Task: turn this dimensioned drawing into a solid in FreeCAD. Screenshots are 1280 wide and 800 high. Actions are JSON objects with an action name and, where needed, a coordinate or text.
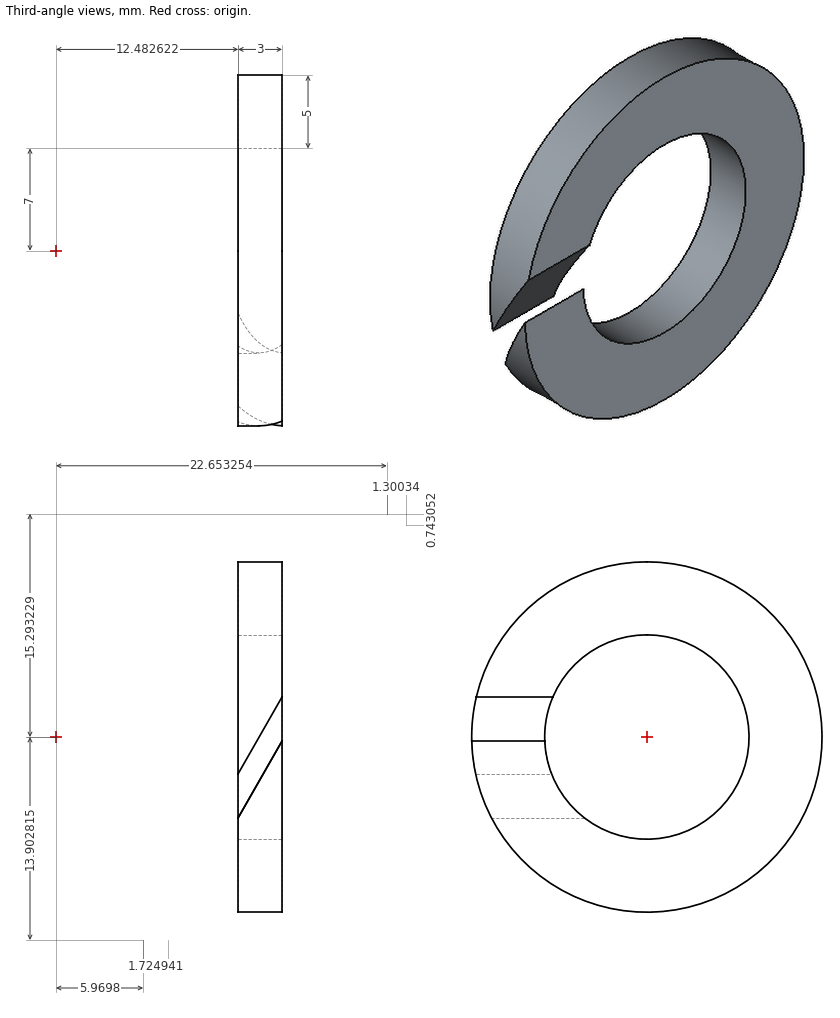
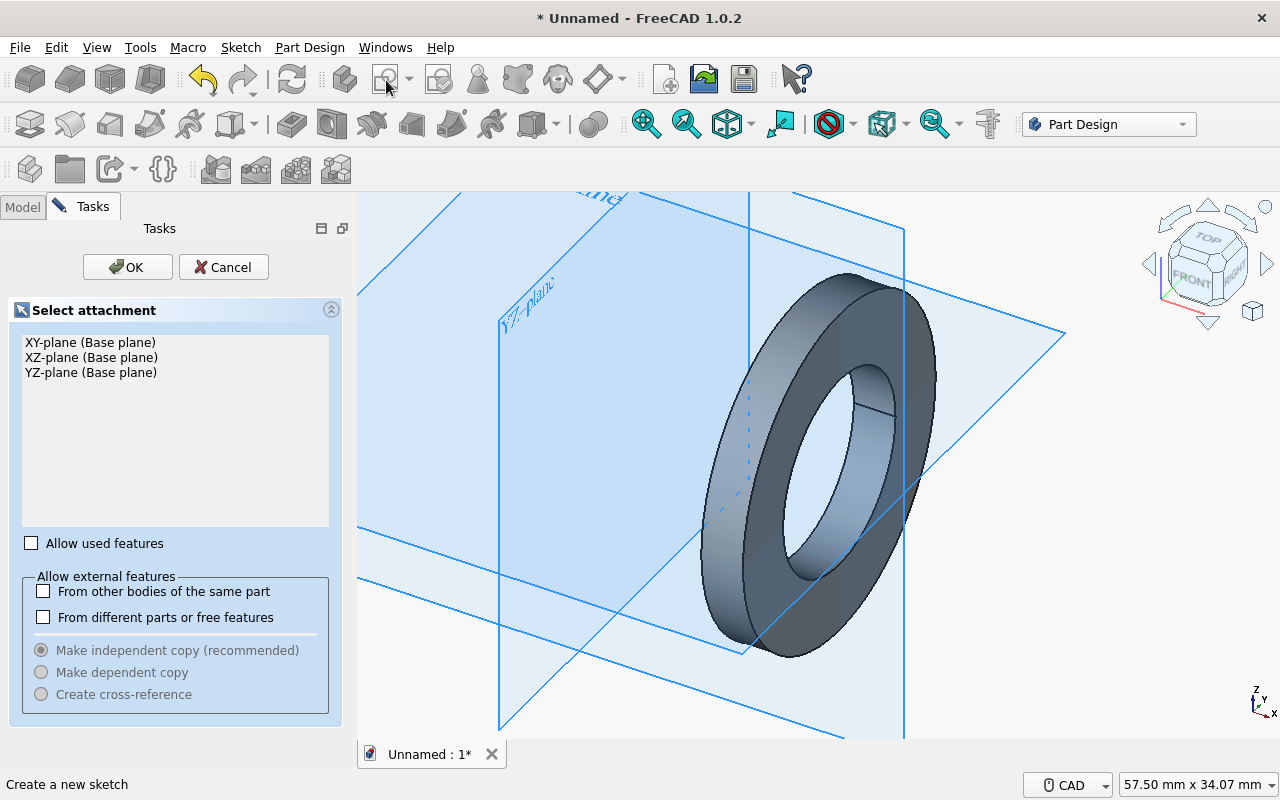
{"action": "left_click", "coordinate": [82, 358]}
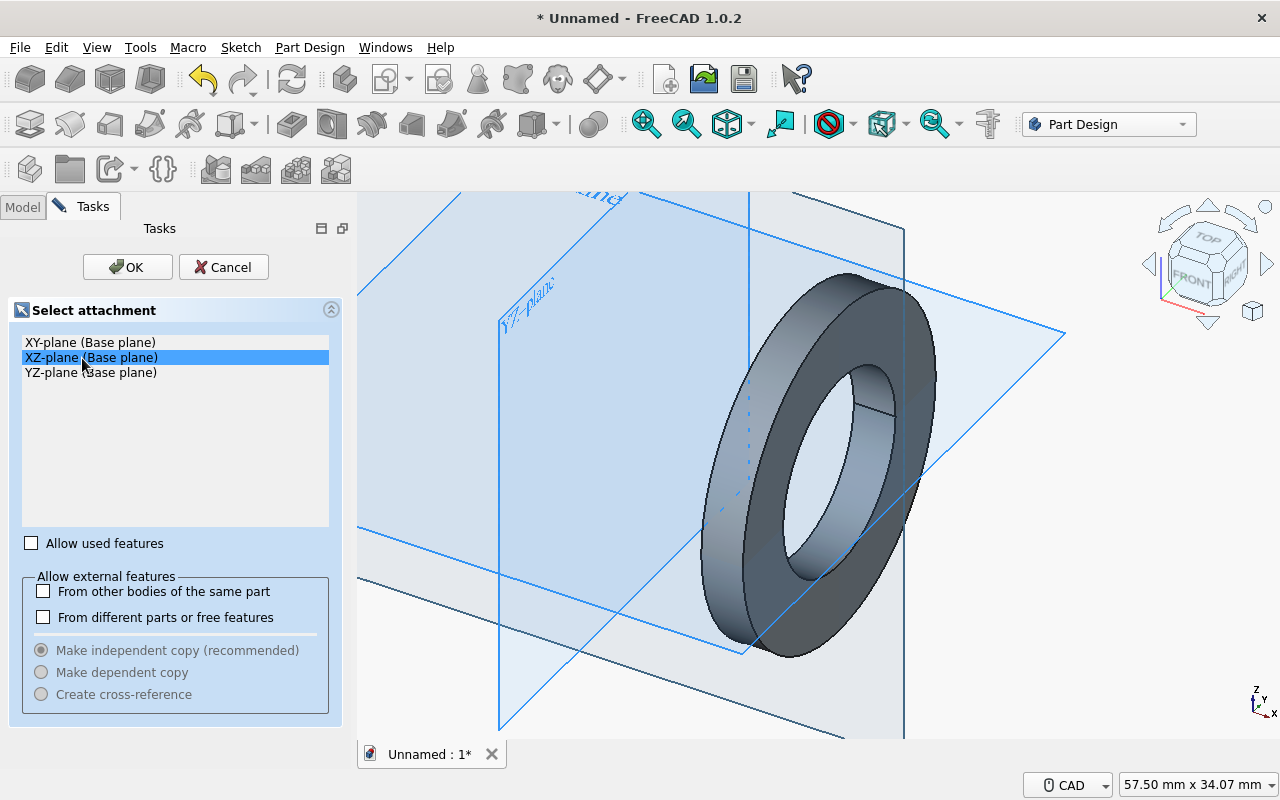
{"action": "left_click", "coordinate": [128, 267]}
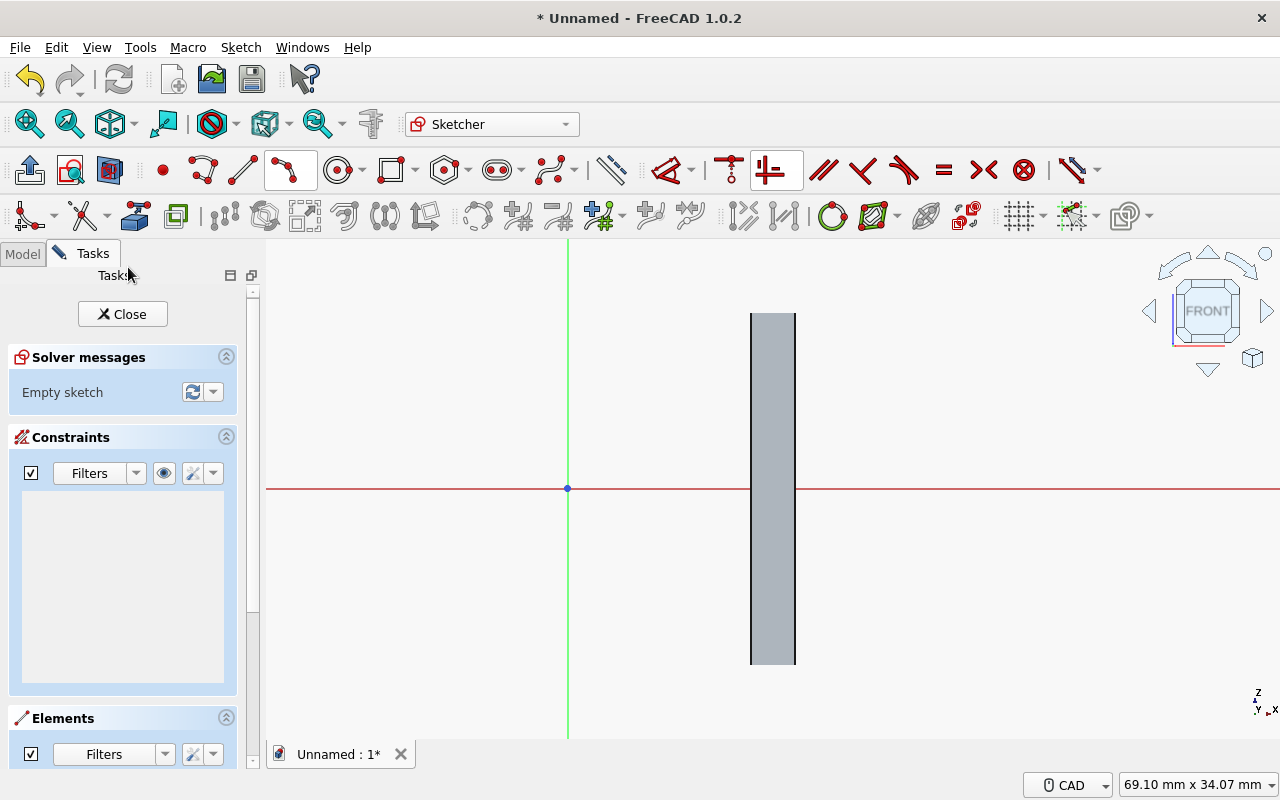
{"action": "key", "text": "q s"}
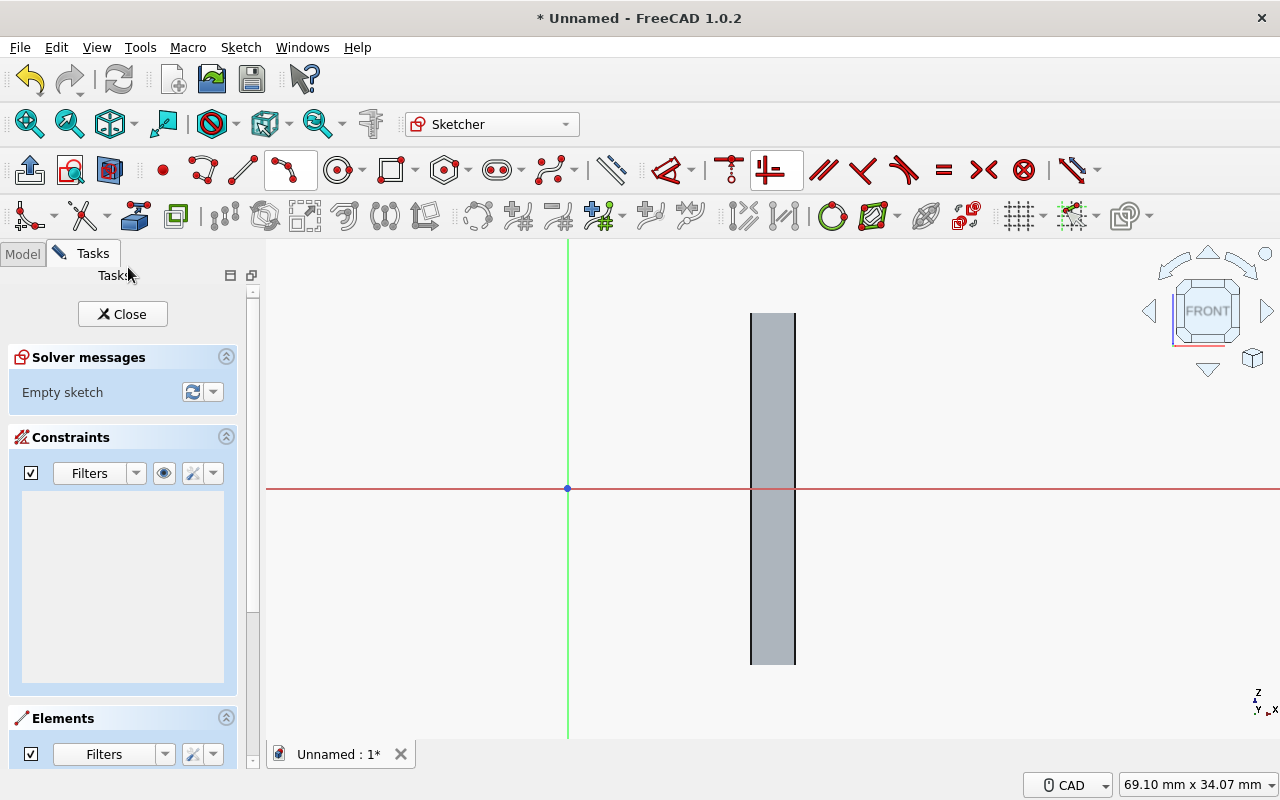
{"action": "scroll", "coordinate": [625, 510], "scroll_direction": "down", "scroll_amount": 2}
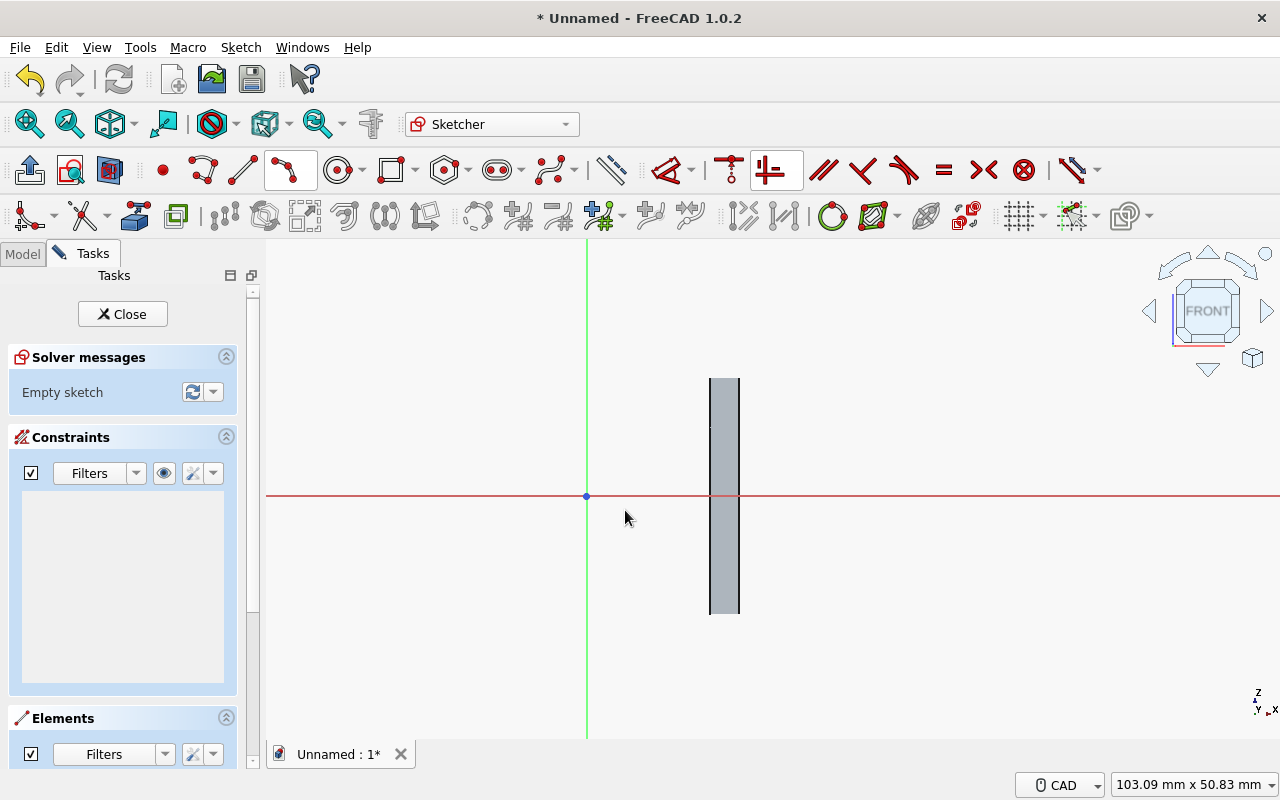
{"action": "key", "text": "g m"}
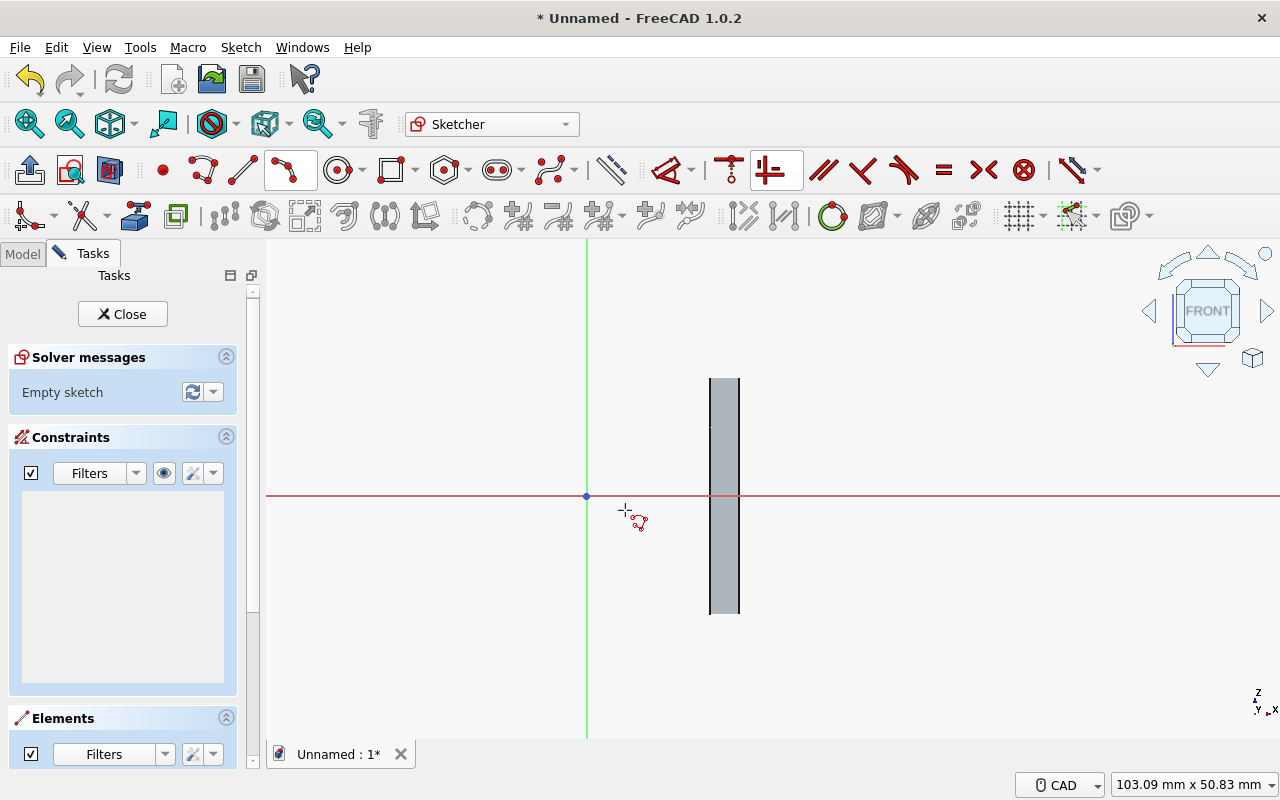
{"action": "left_click", "coordinate": [646, 633]}
{"action": "left_click", "coordinate": [810, 346]}
{"action": "left_click", "coordinate": [822, 353]}
{"action": "left_click", "coordinate": [662, 633]}
{"action": "left_click", "coordinate": [646, 634]}
{"action": "key", "text": "Escape"}
{"action": "key", "text": "Escape"}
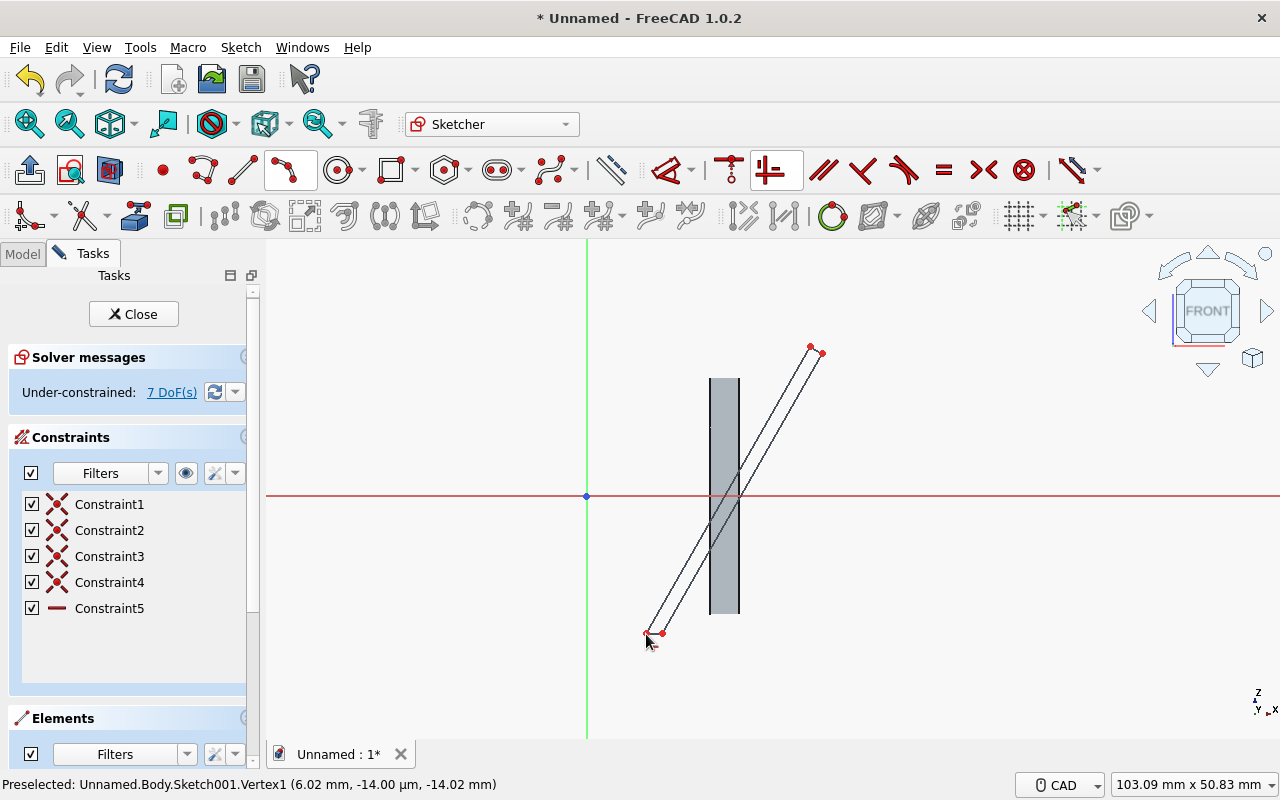
{"action": "key", "text": "d"}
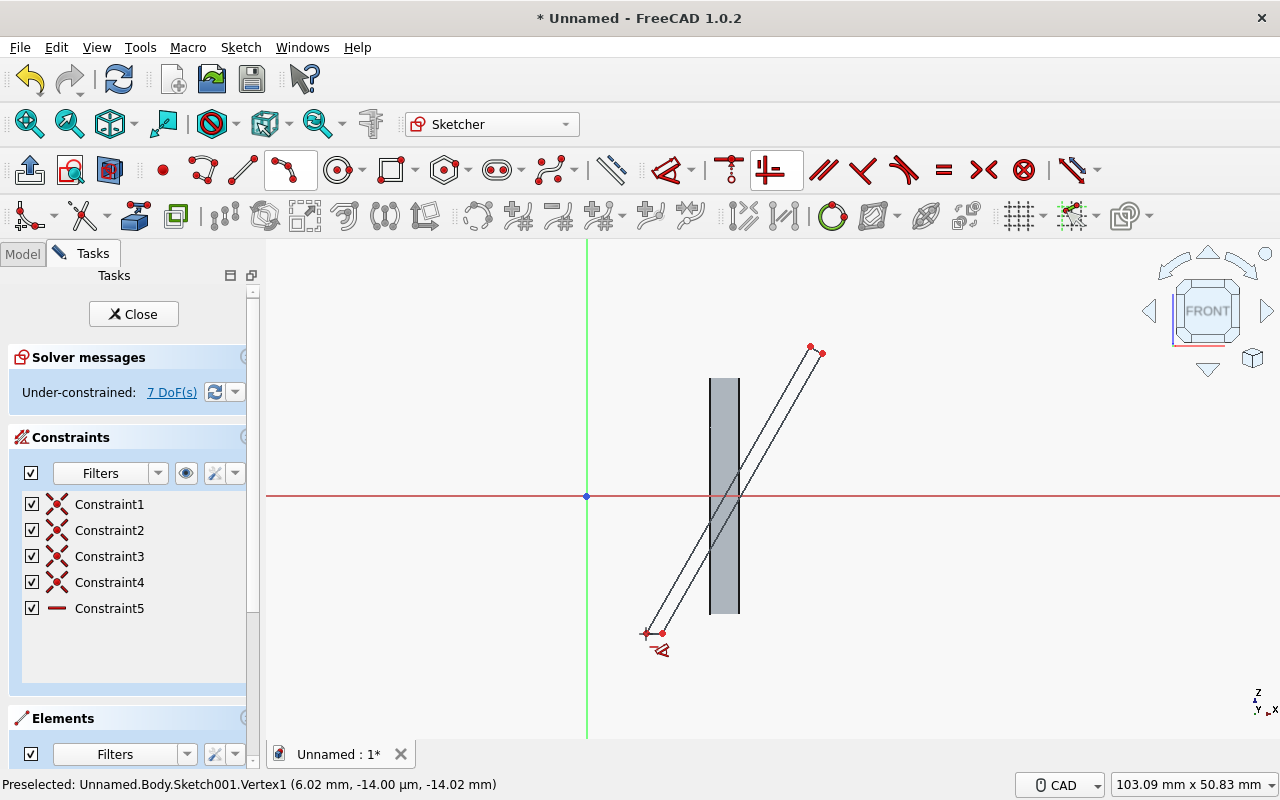
{"action": "left_click", "coordinate": [646, 634]}
{"action": "left_click", "coordinate": [616, 668]}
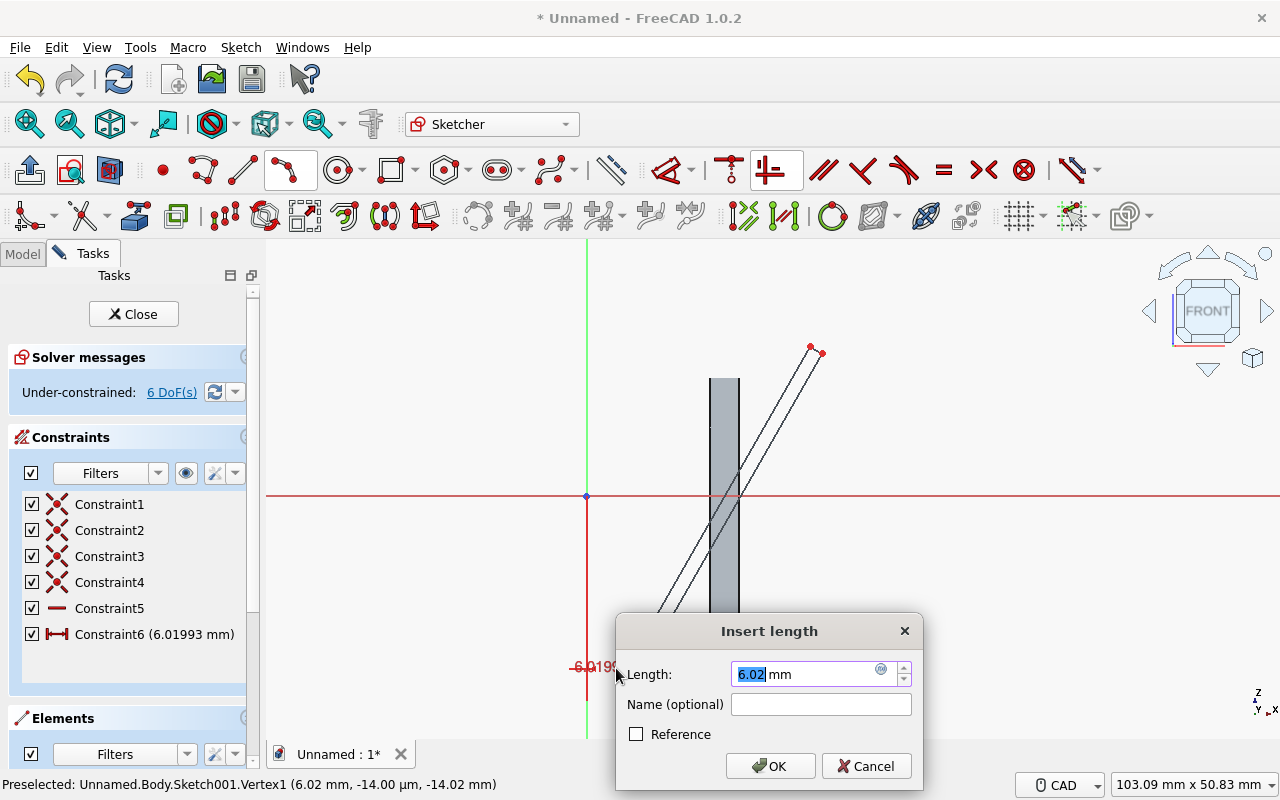
{"action": "type", "text": "5.9698"}
{"action": "key", "text": "Return"}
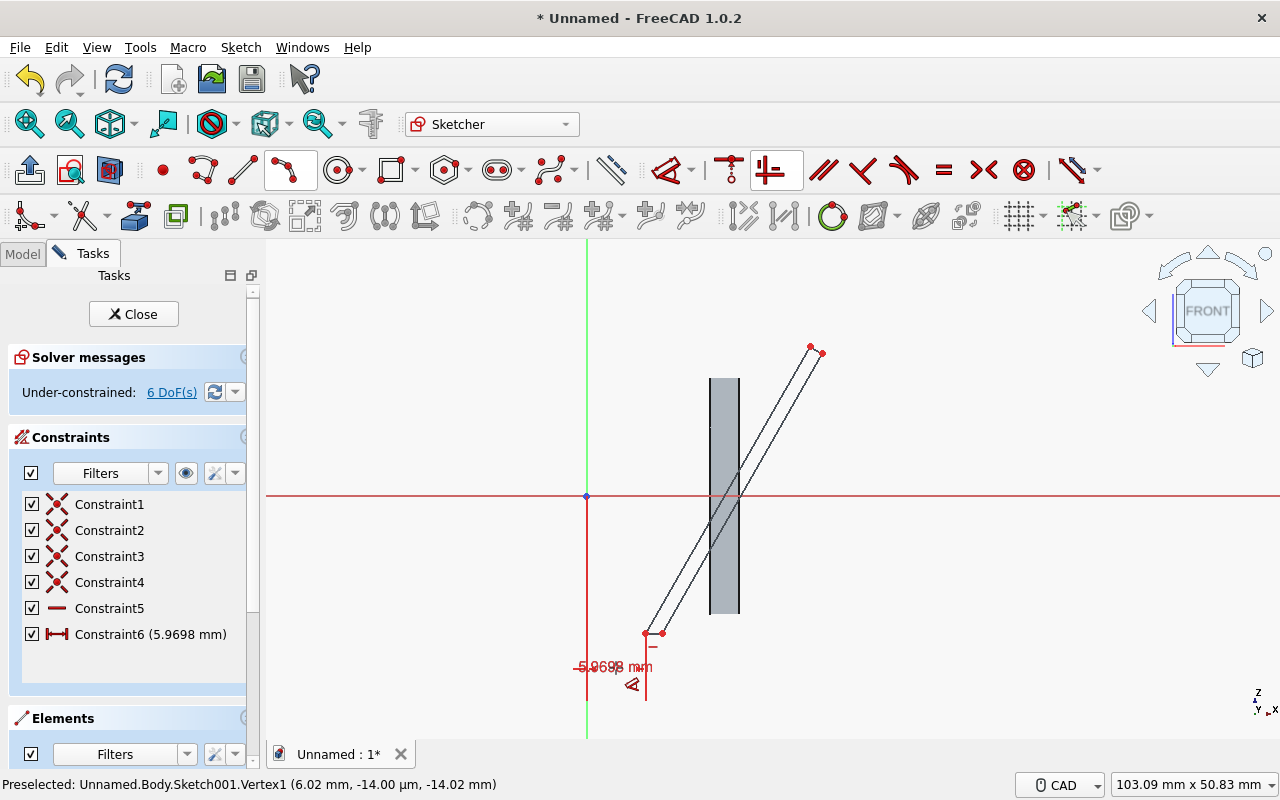
{"action": "scroll", "coordinate": [654, 634], "scroll_direction": "up", "scroll_amount": 5}